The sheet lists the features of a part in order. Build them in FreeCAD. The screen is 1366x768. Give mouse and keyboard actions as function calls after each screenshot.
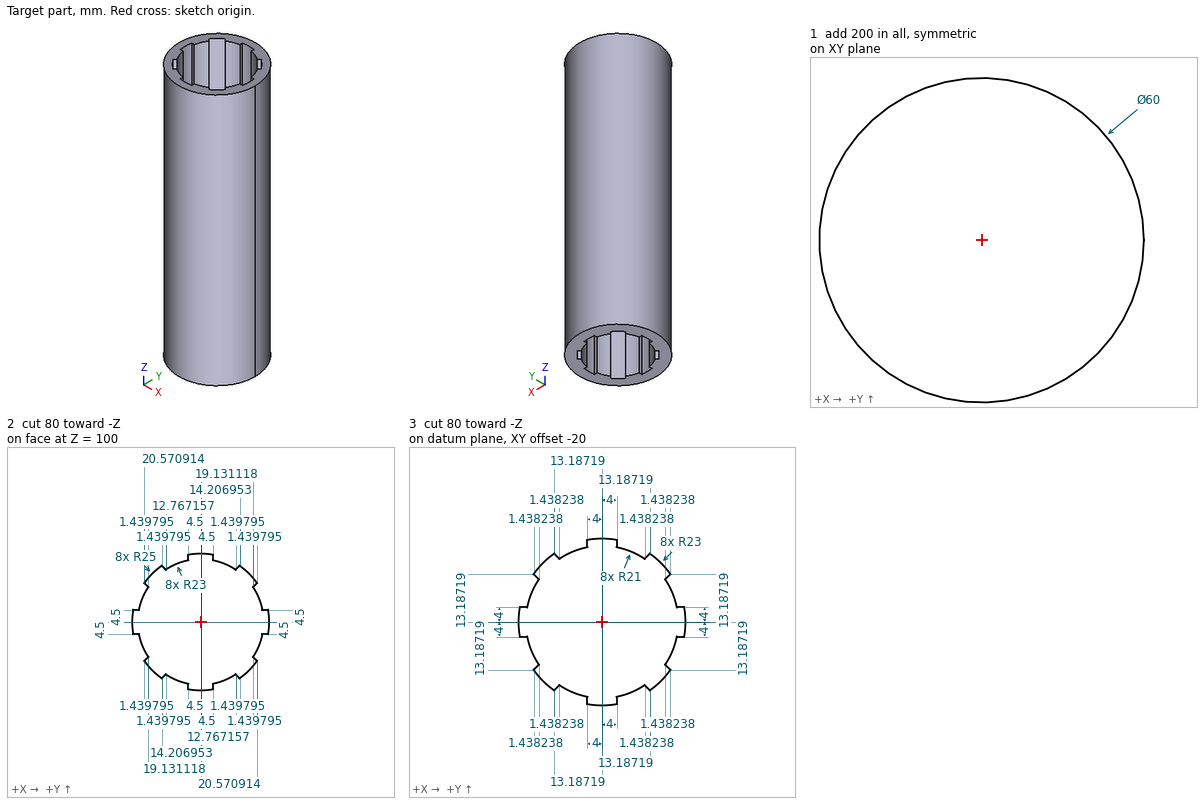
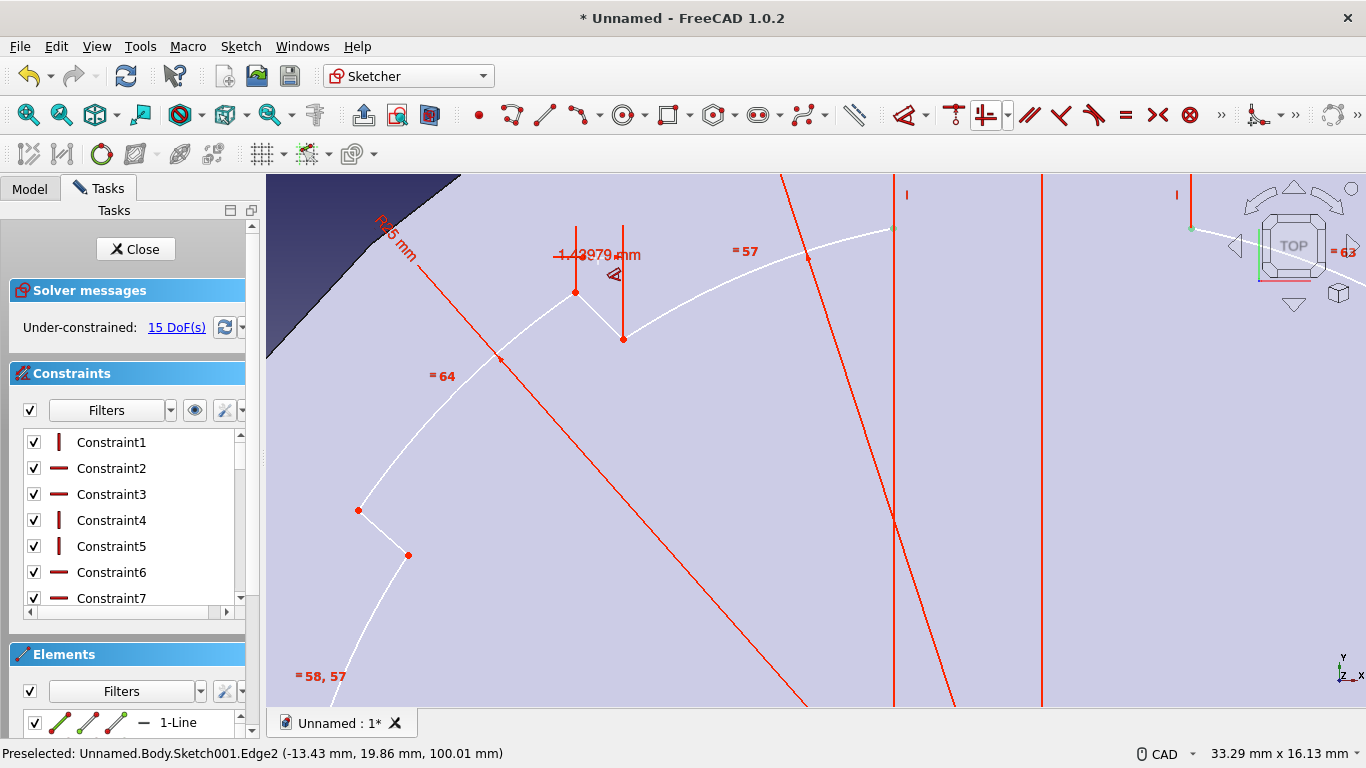
click(373, 524)
click(366, 477)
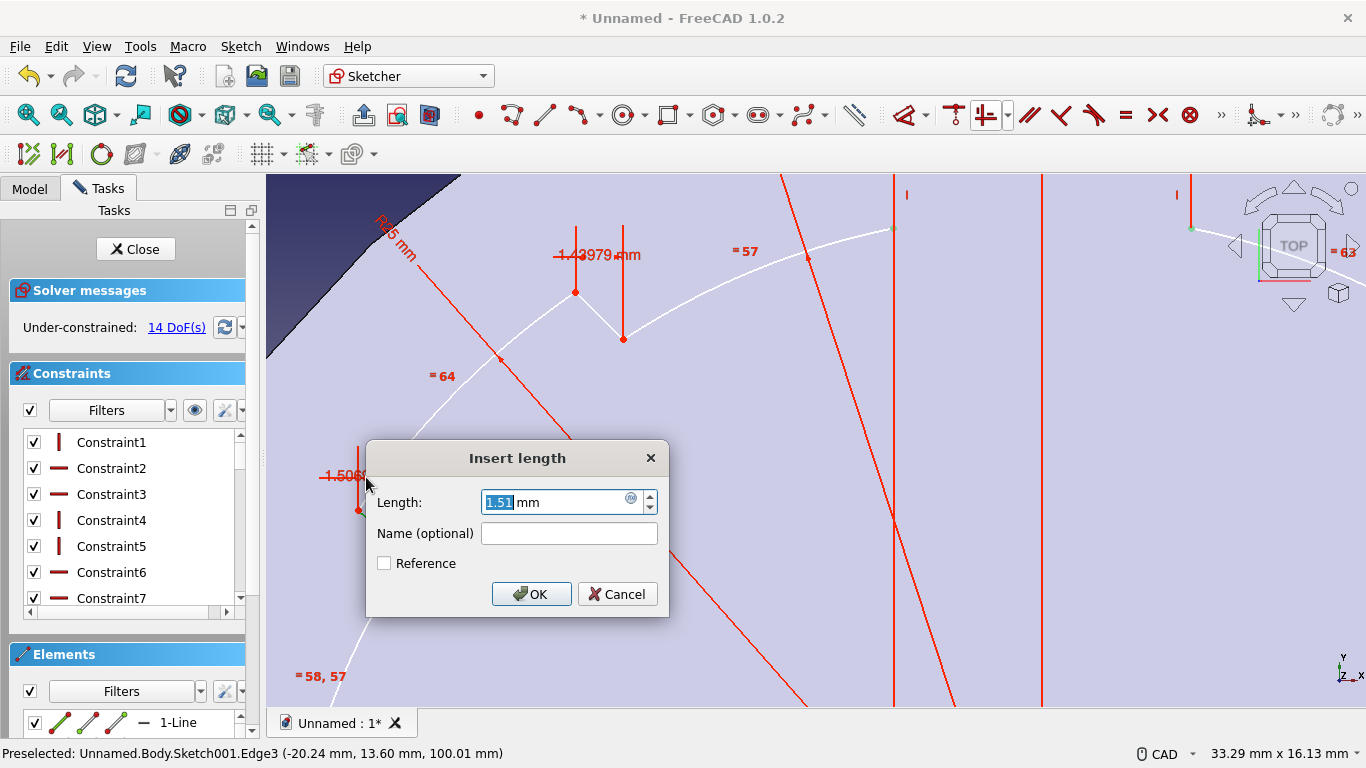
text(1.439795)
key(Return)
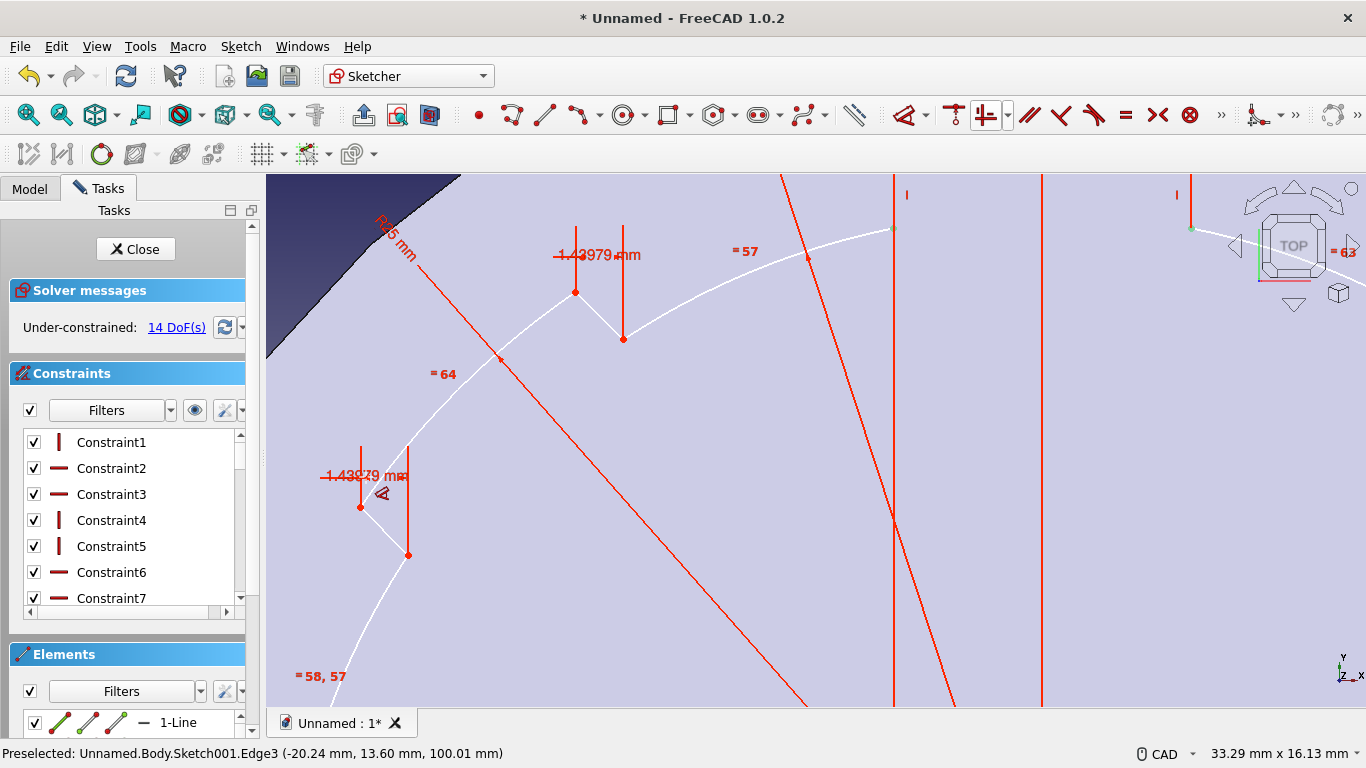
scroll(673, 306, down, 8)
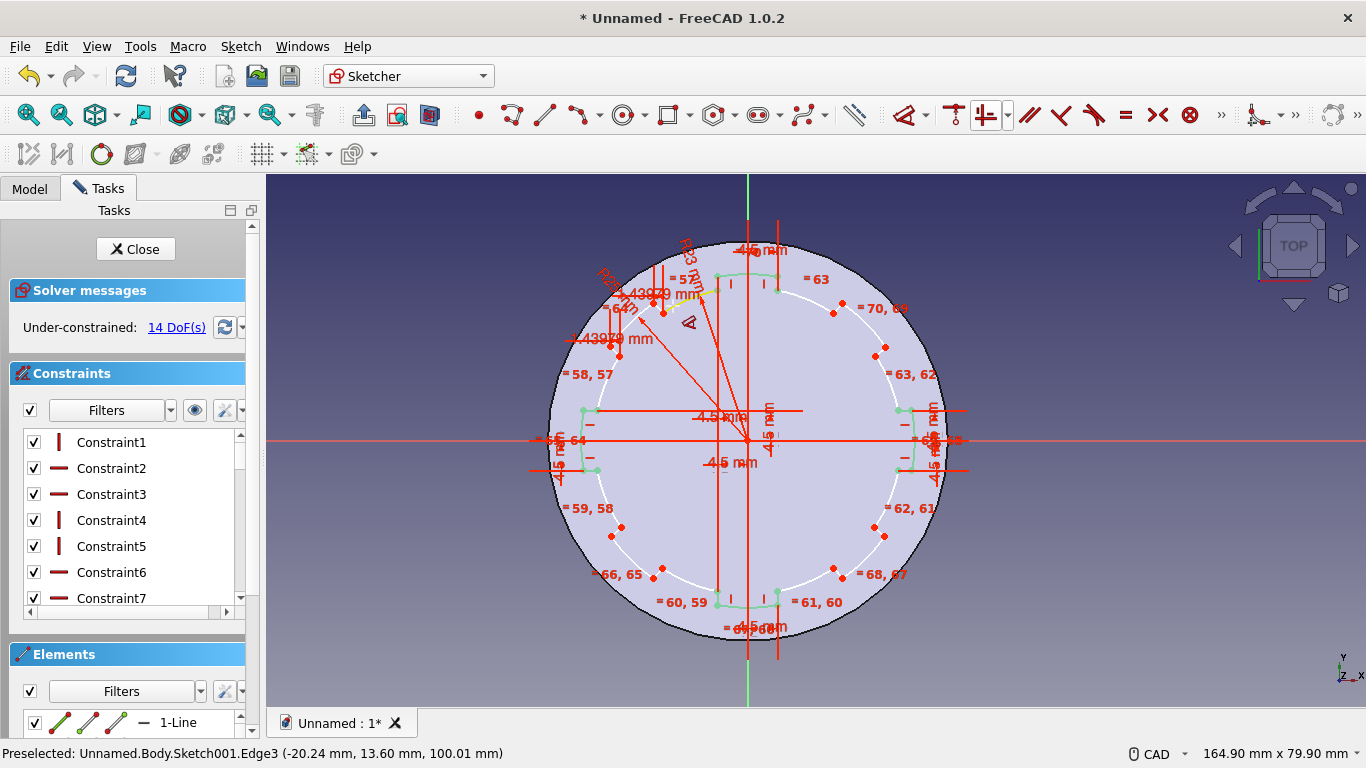
scroll(618, 530, up, 8)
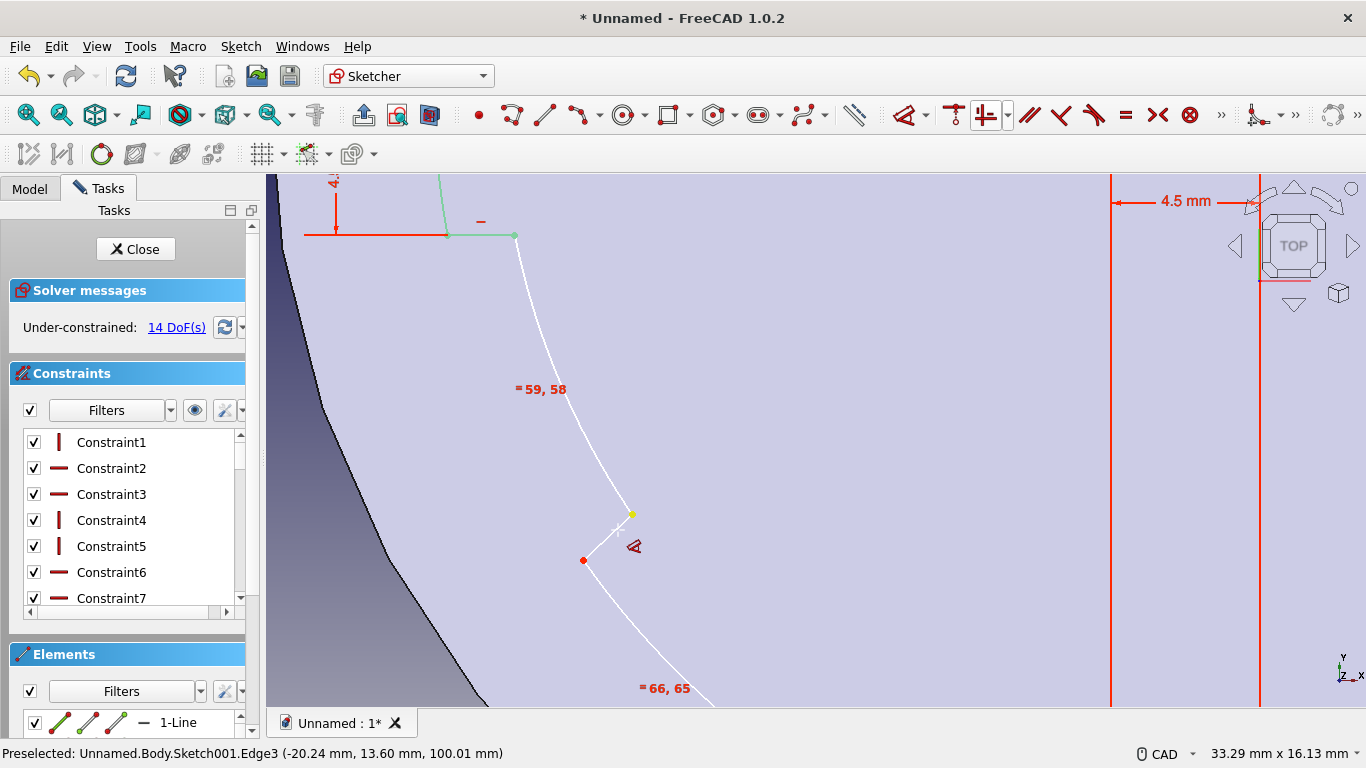
click(618, 528)
click(591, 594)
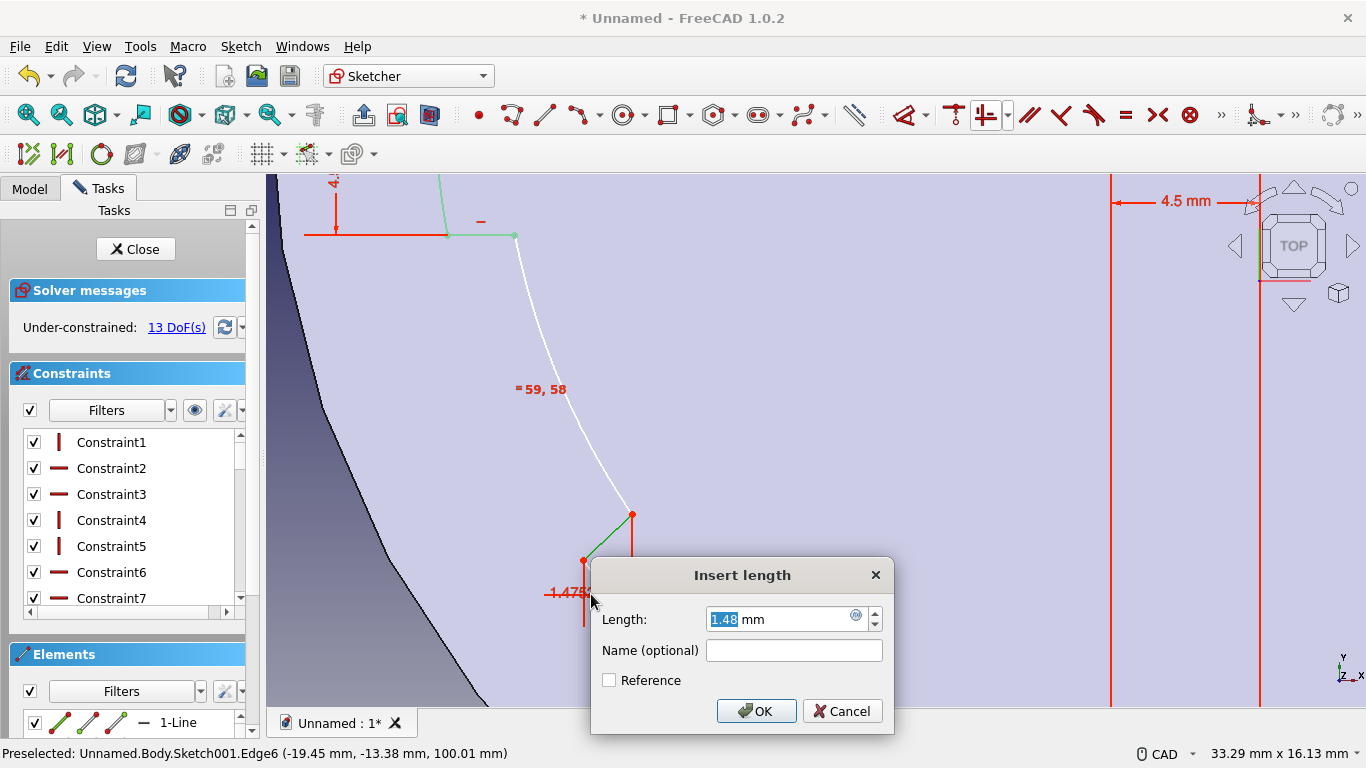
text(1.439795)
key(Return)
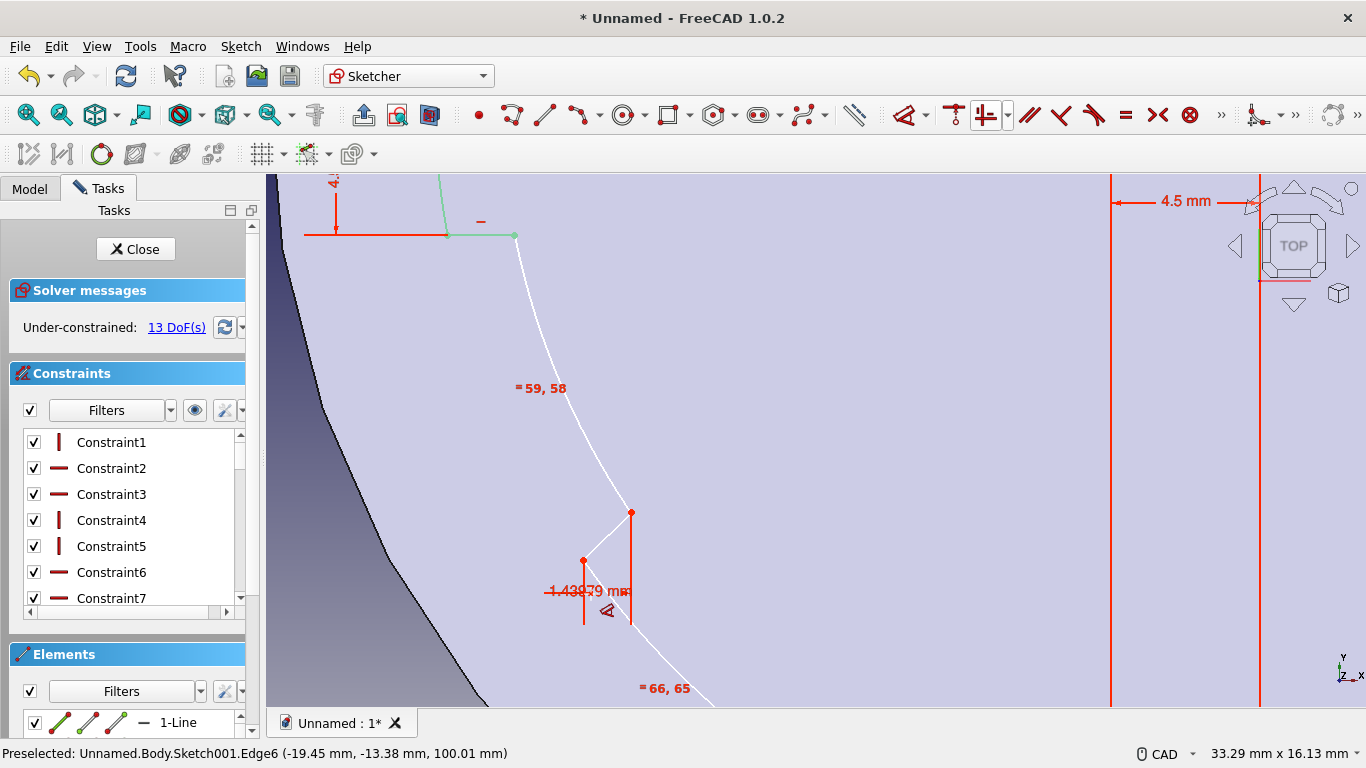
scroll(618, 530, down, 8)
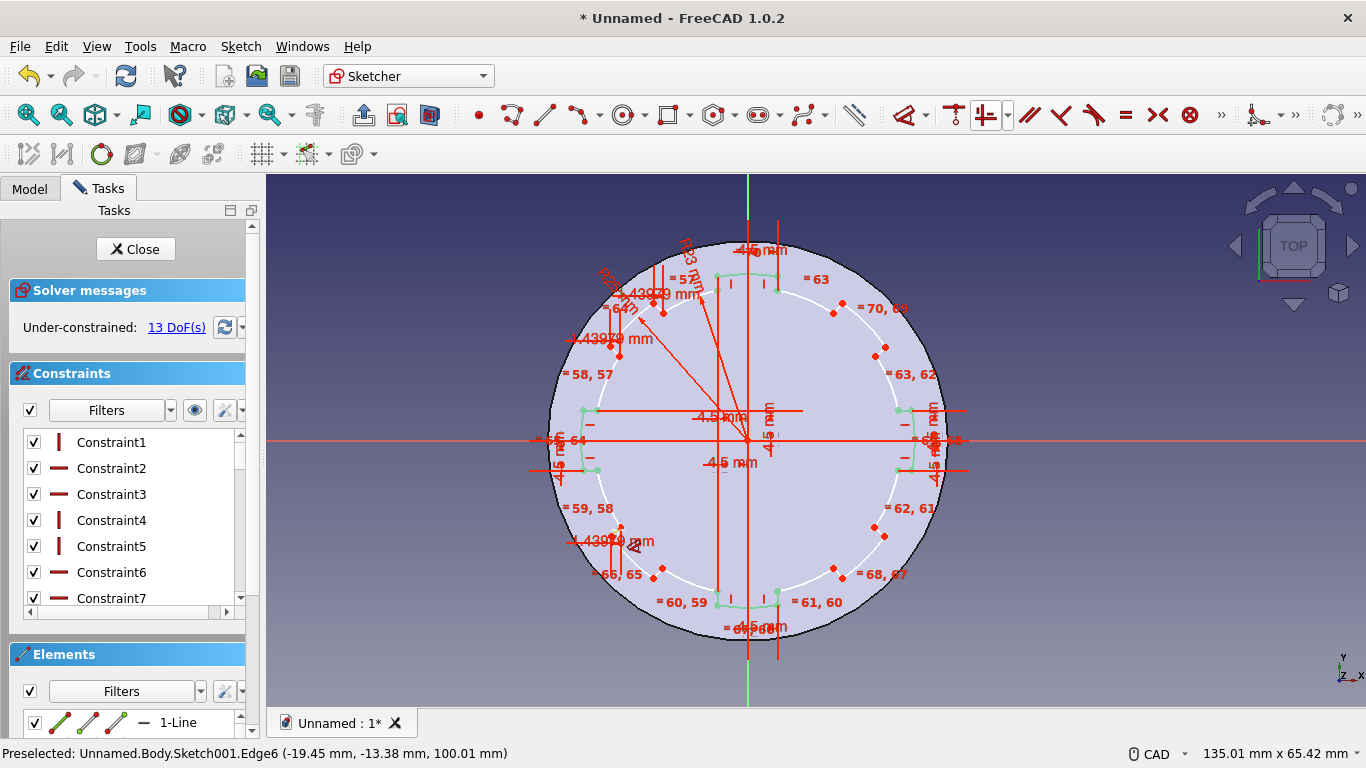
scroll(656, 575, up, 8)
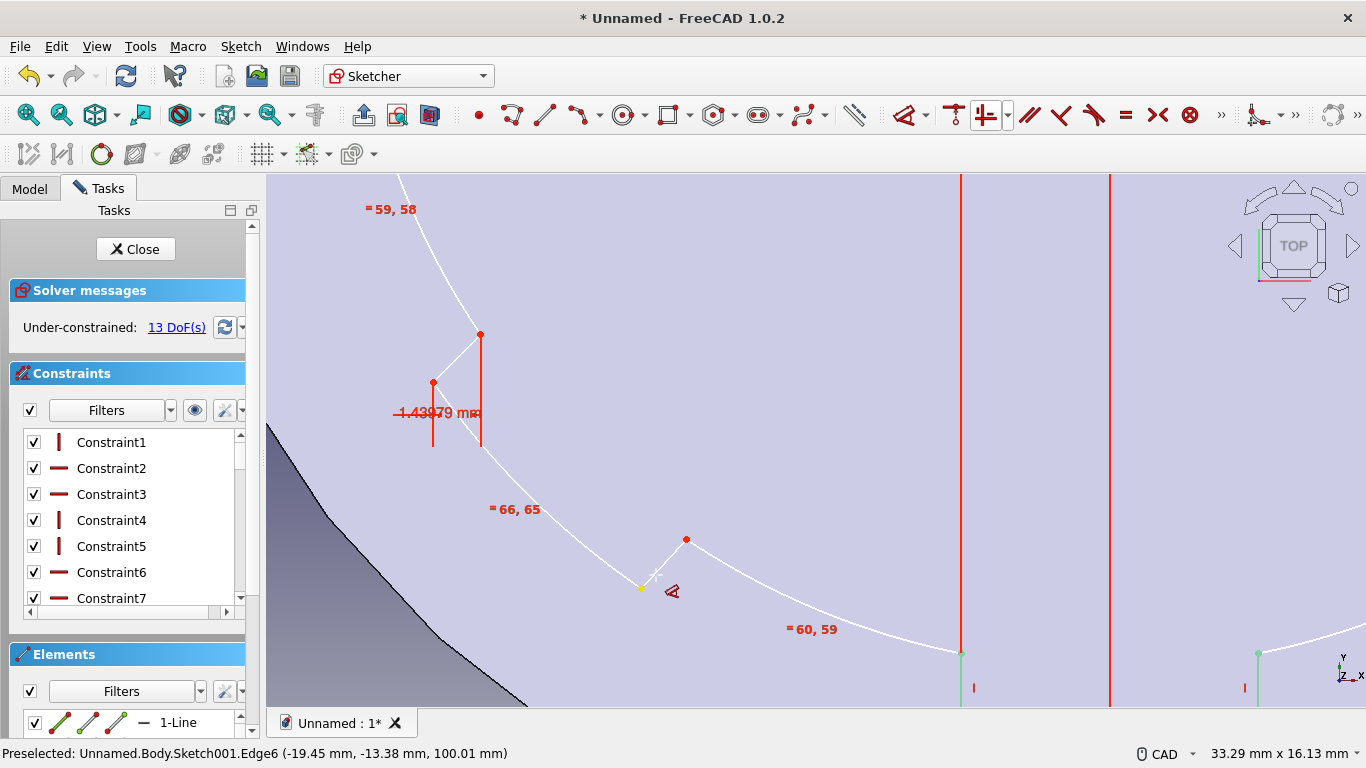
click(655, 574)
click(664, 623)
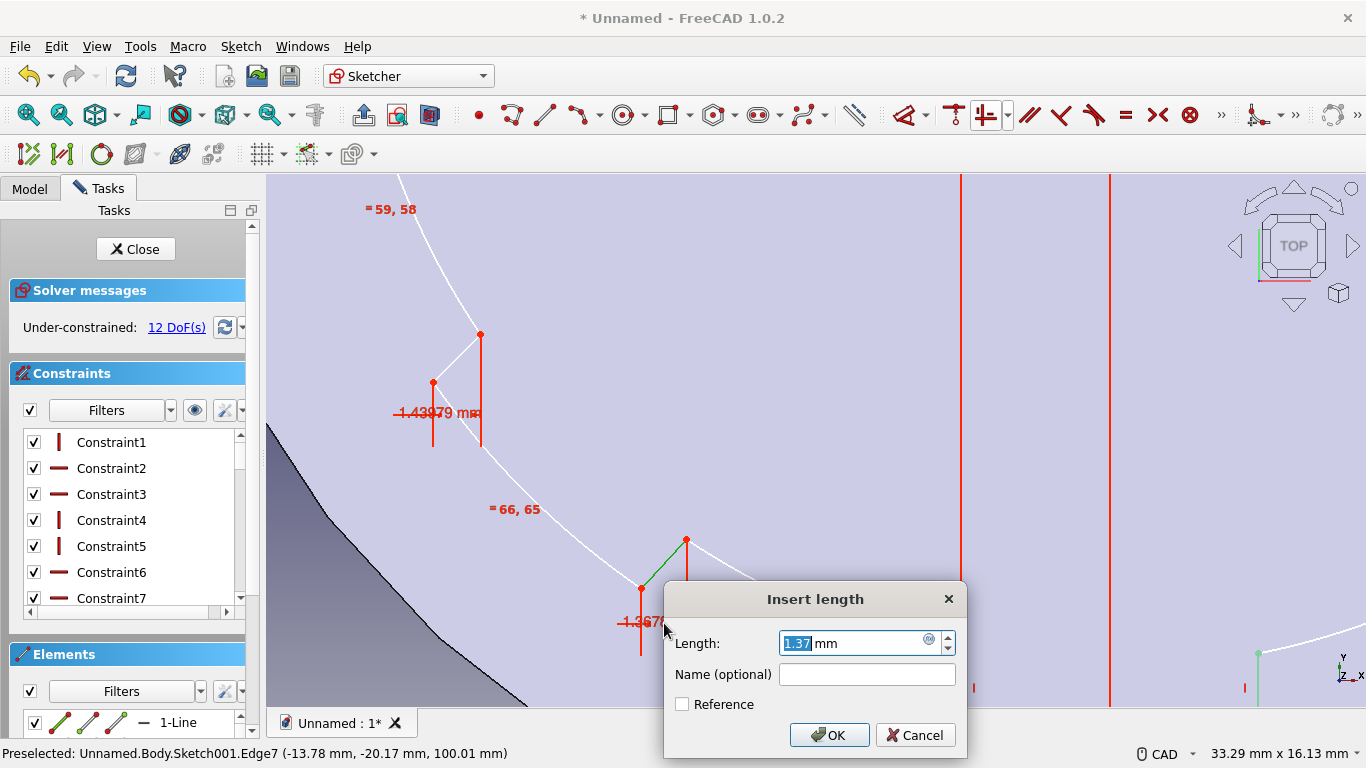
text(1.439795)
key(Return)